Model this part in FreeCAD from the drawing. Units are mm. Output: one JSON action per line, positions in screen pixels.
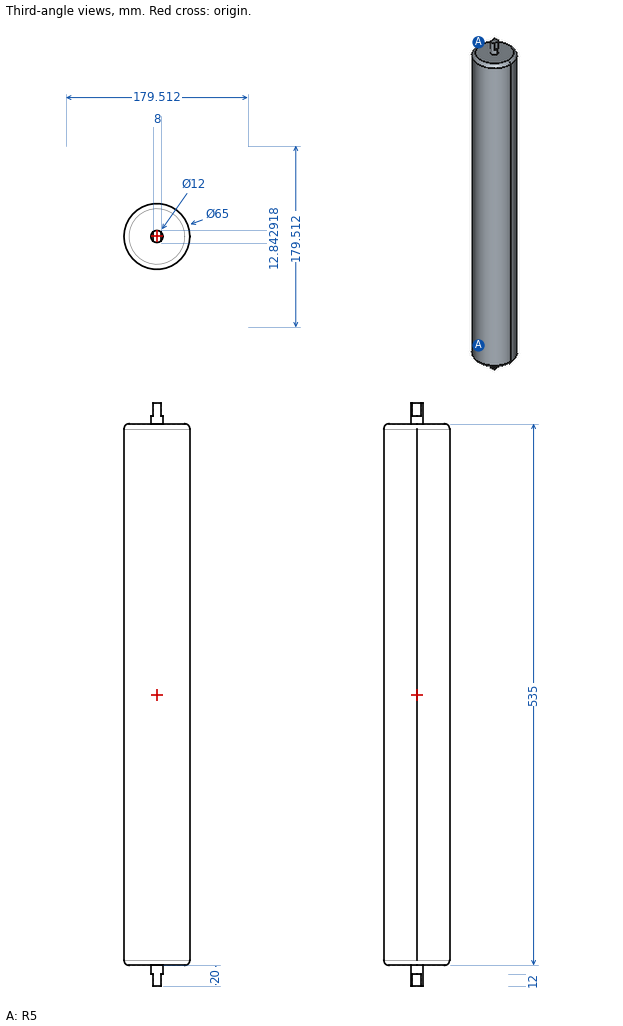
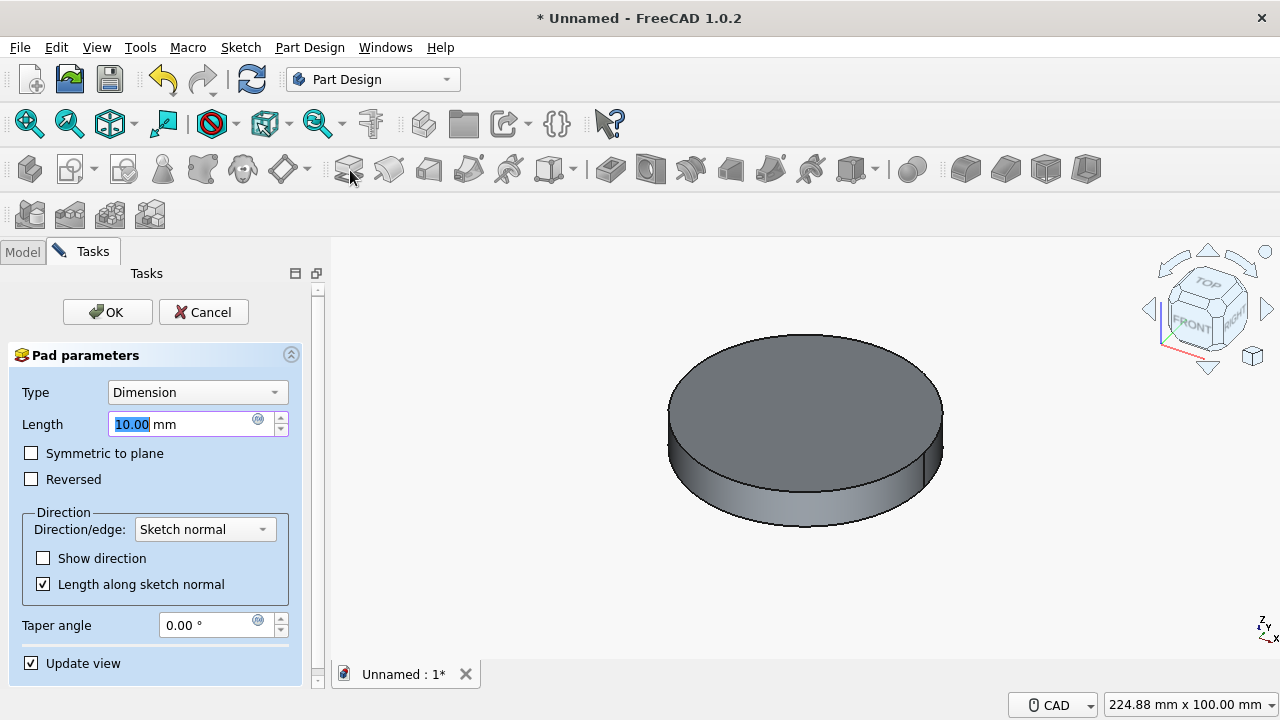
{"action": "type", "text": "535"}
{"action": "key", "text": "Tab"}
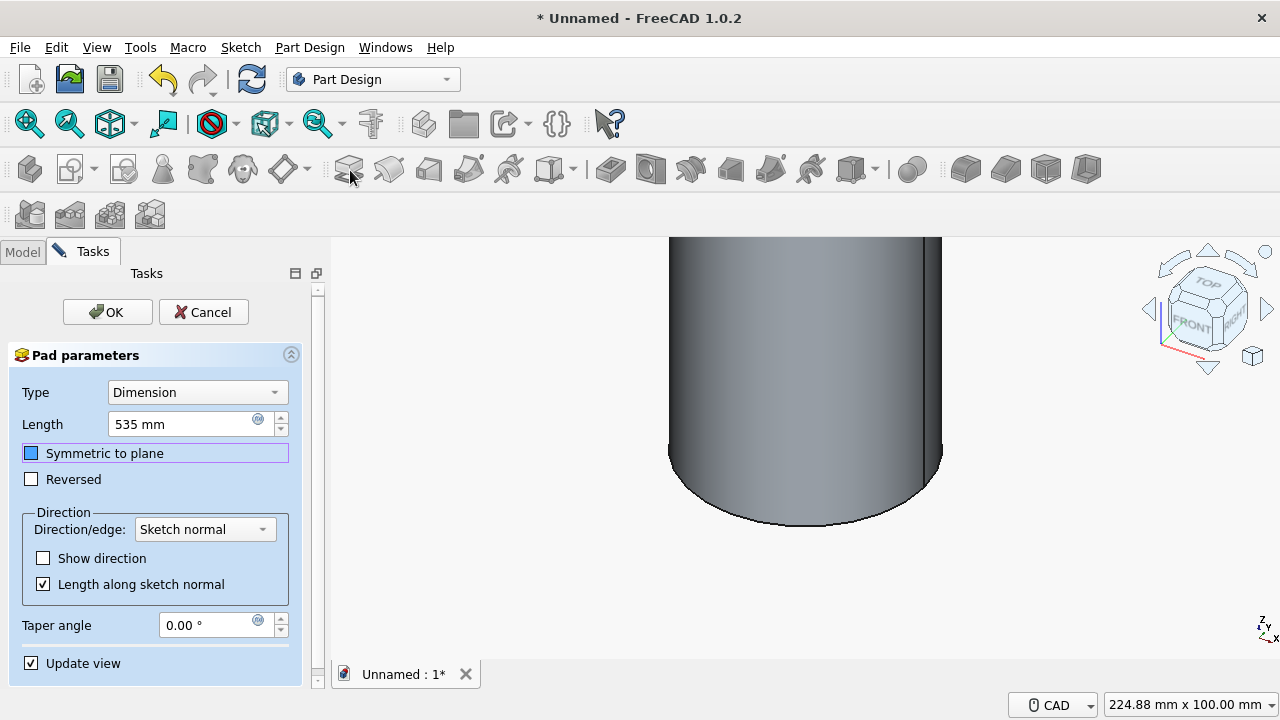
{"action": "left_click", "coordinate": [30, 453]}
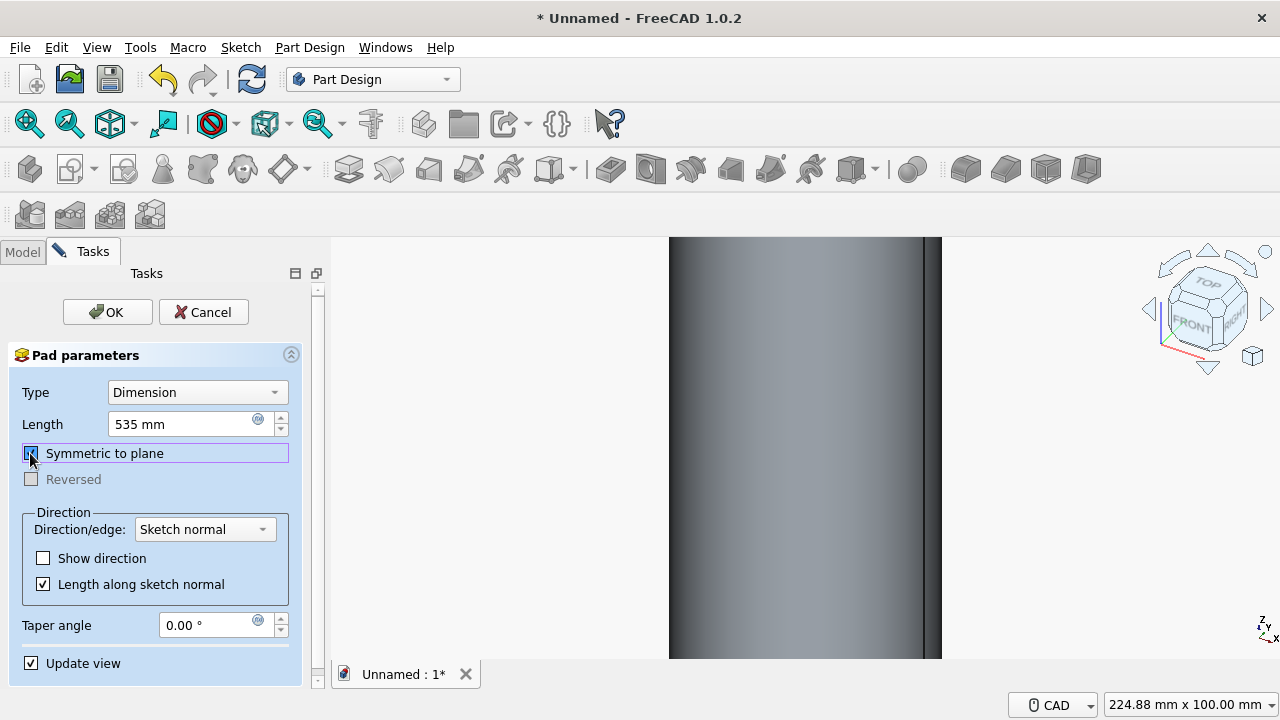
{"action": "left_click", "coordinate": [108, 312]}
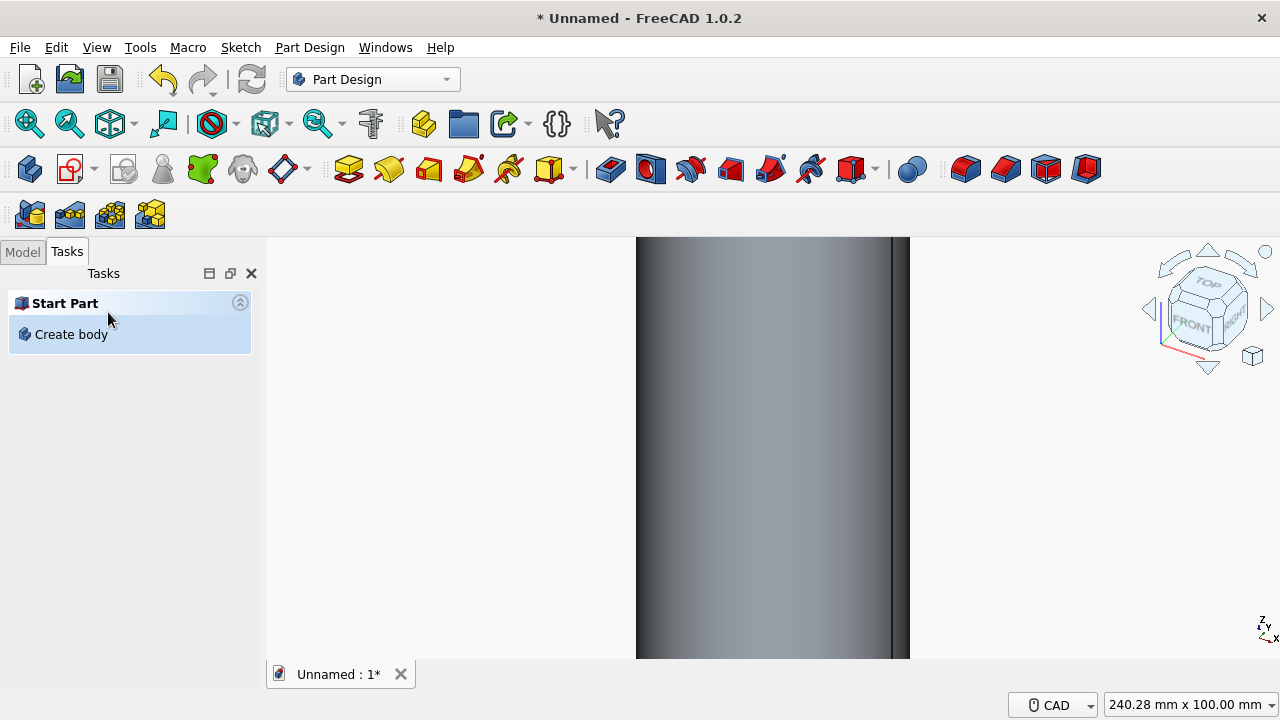
{"action": "left_click", "coordinate": [30, 124]}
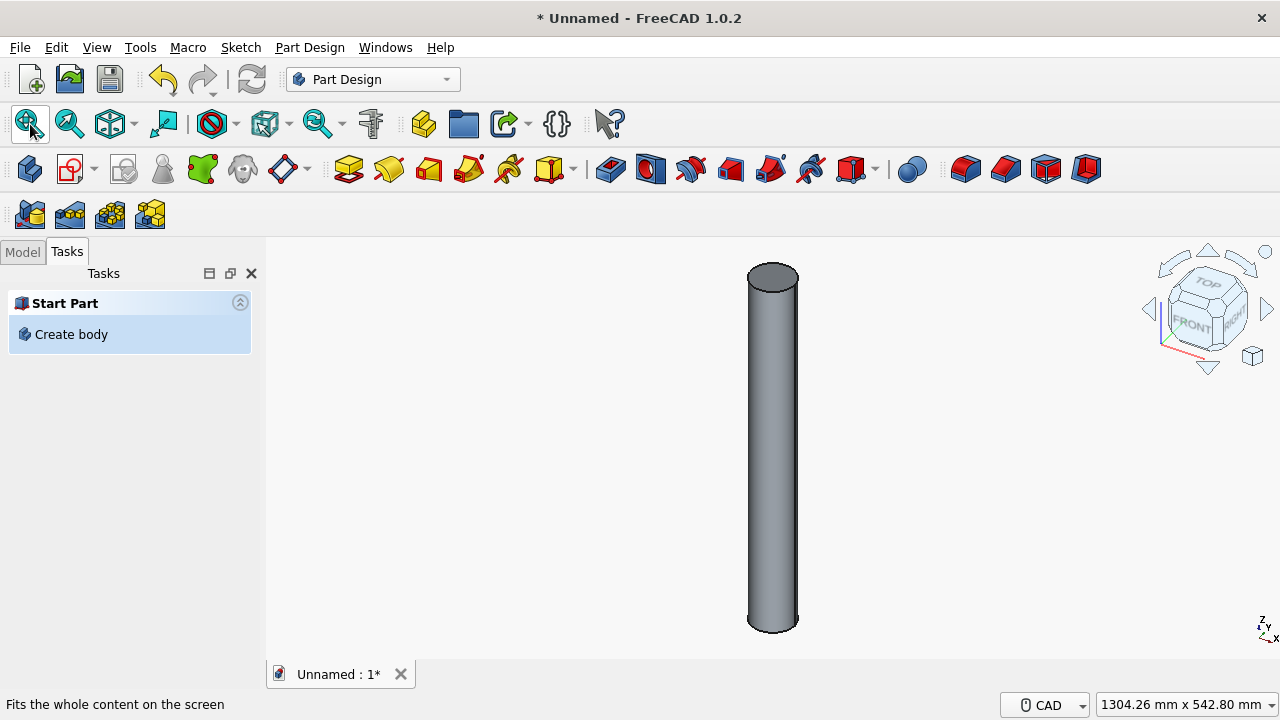
{"action": "key", "text": "5"}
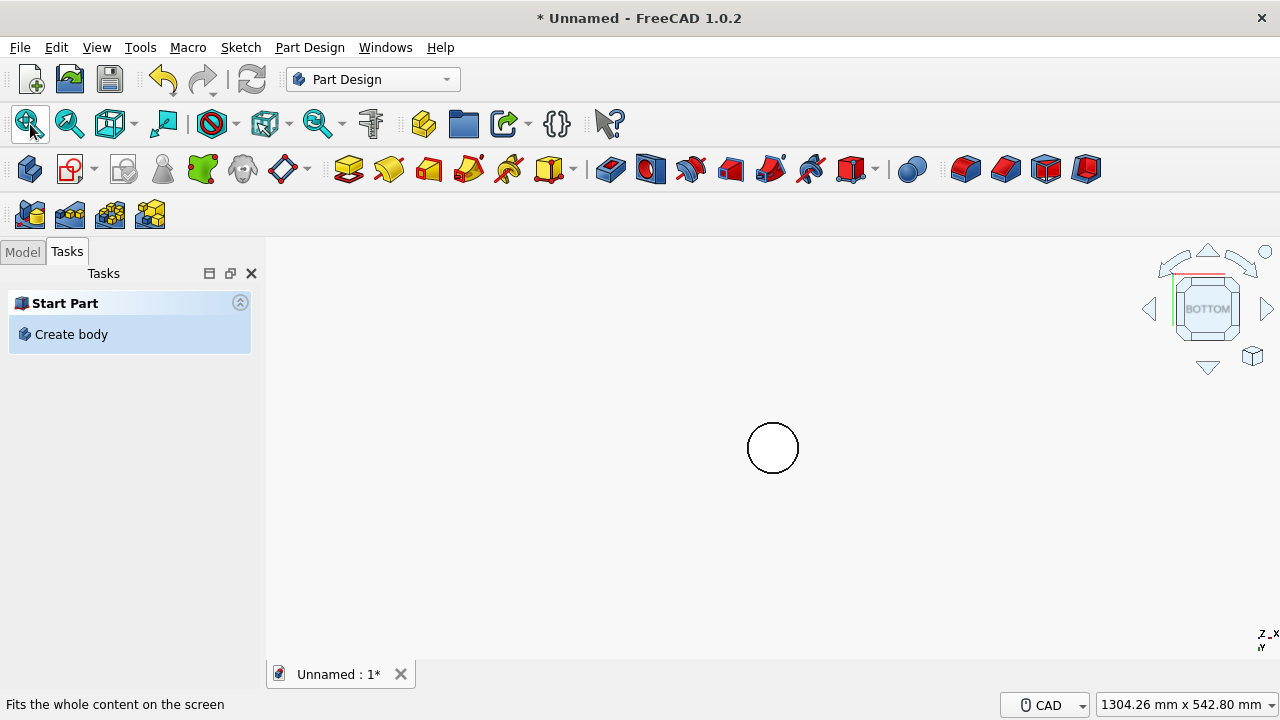
{"action": "left_click", "coordinate": [30, 124]}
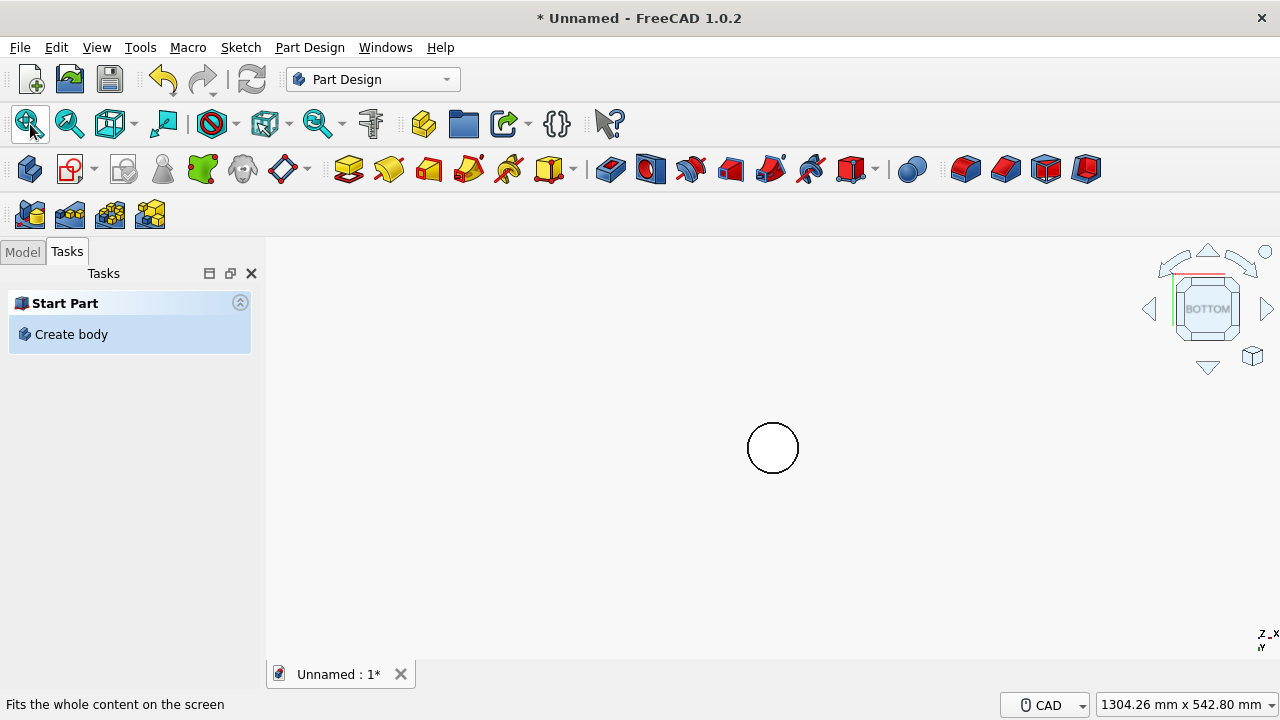
{"action": "left_click", "coordinate": [773, 447]}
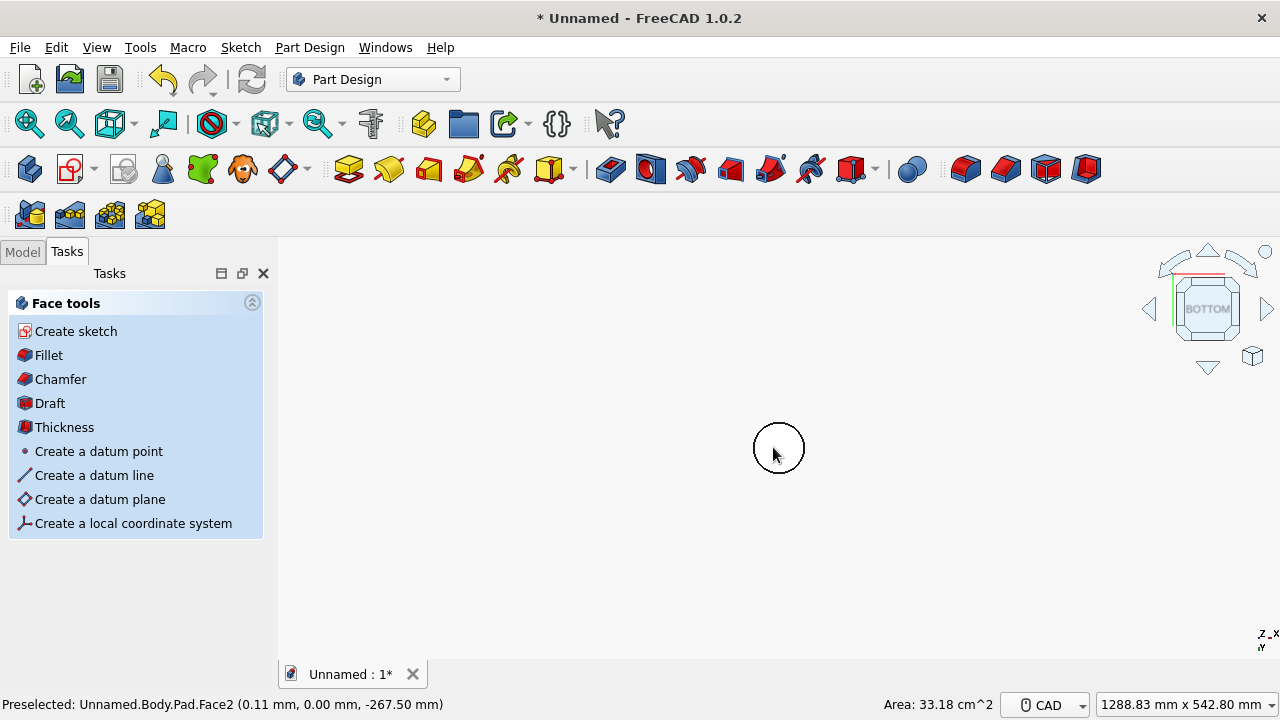
{"action": "left_click", "coordinate": [70, 170]}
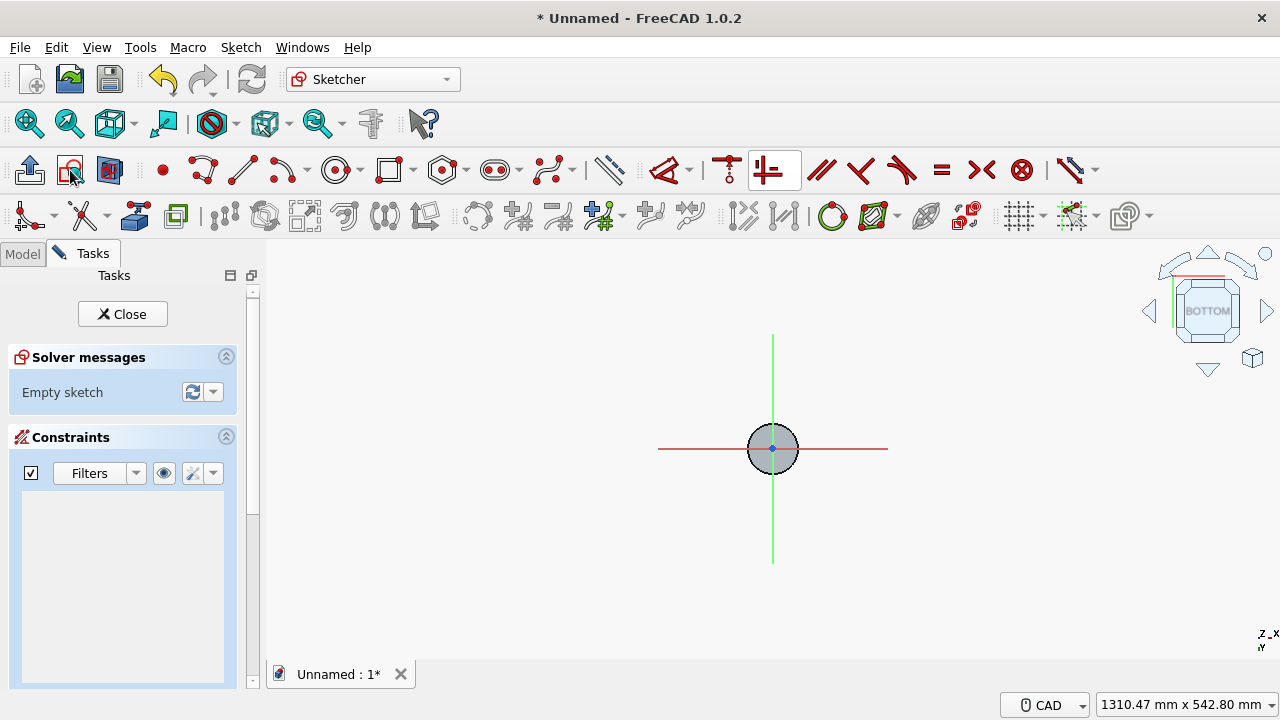
{"action": "scroll", "coordinate": [776, 449], "scroll_direction": "up", "scroll_amount": 15}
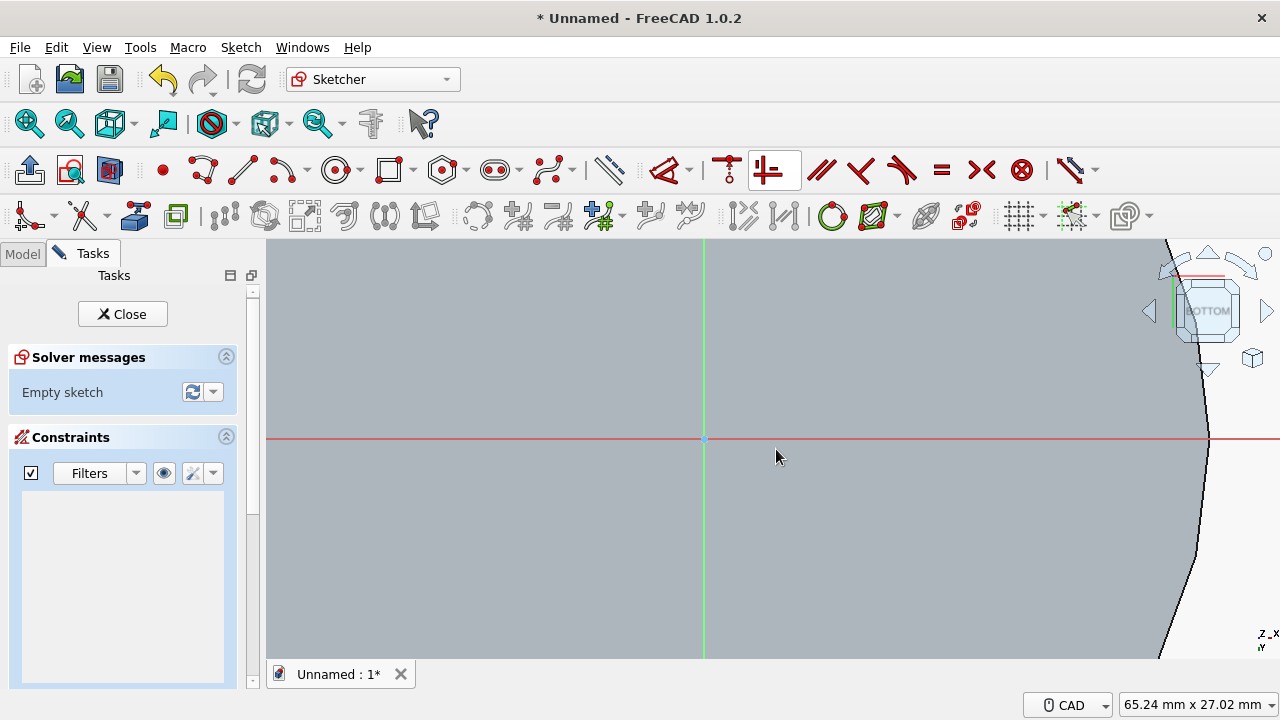
{"action": "scroll", "coordinate": [704, 420], "scroll_direction": "up", "scroll_amount": 2}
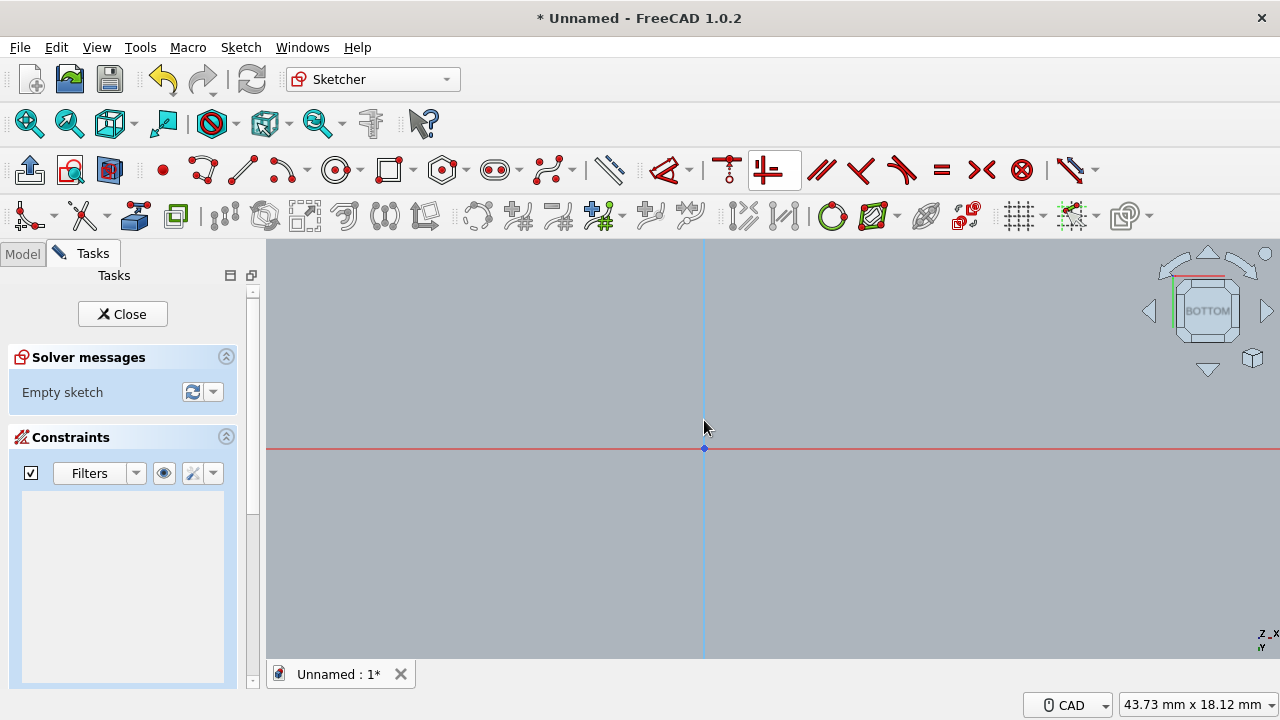
{"action": "left_click", "coordinate": [336, 170]}